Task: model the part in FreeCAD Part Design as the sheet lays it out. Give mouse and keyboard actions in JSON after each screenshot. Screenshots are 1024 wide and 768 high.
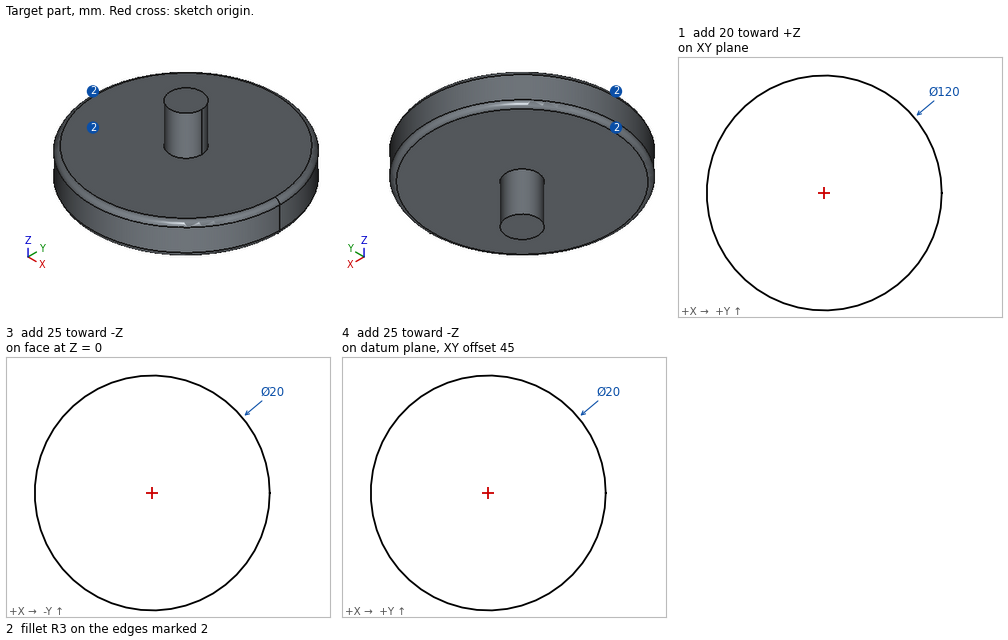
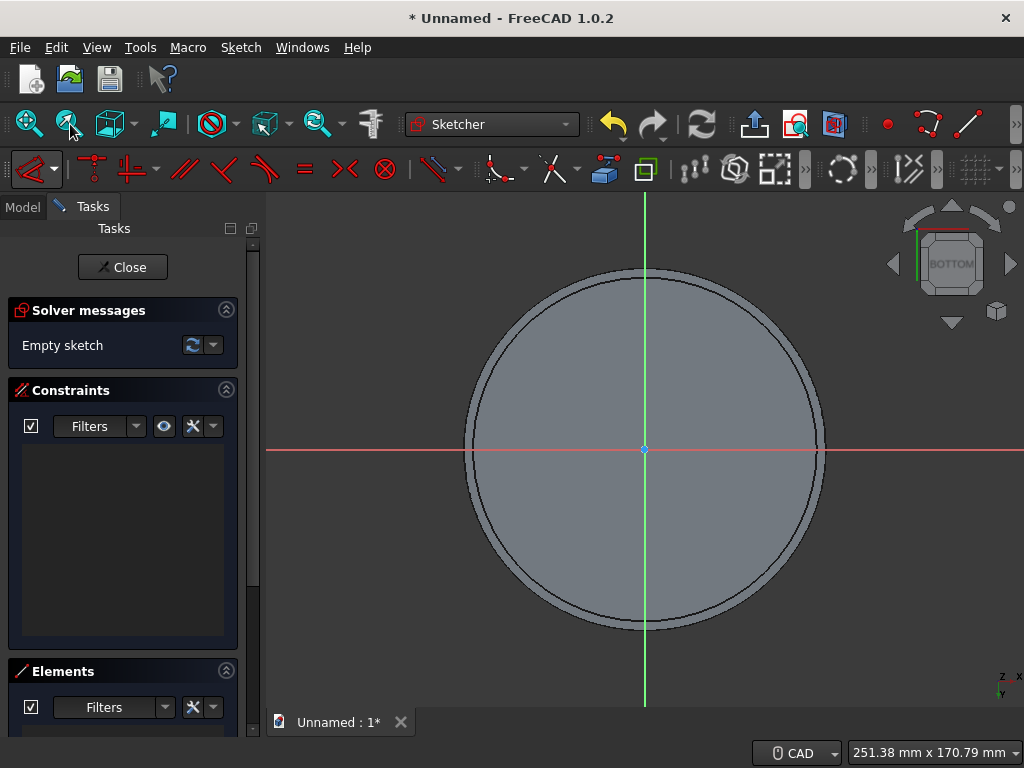
{"action": "scroll", "coordinate": [662, 449], "scroll_direction": "up", "scroll_amount": 8}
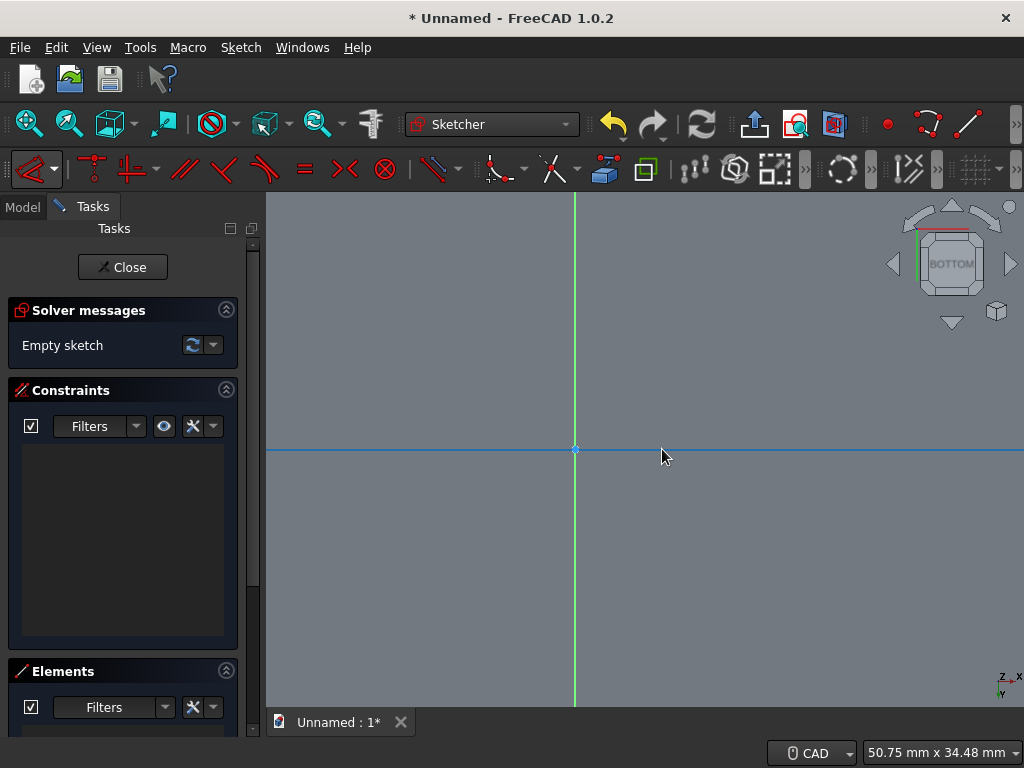
{"action": "key", "text": "g c"}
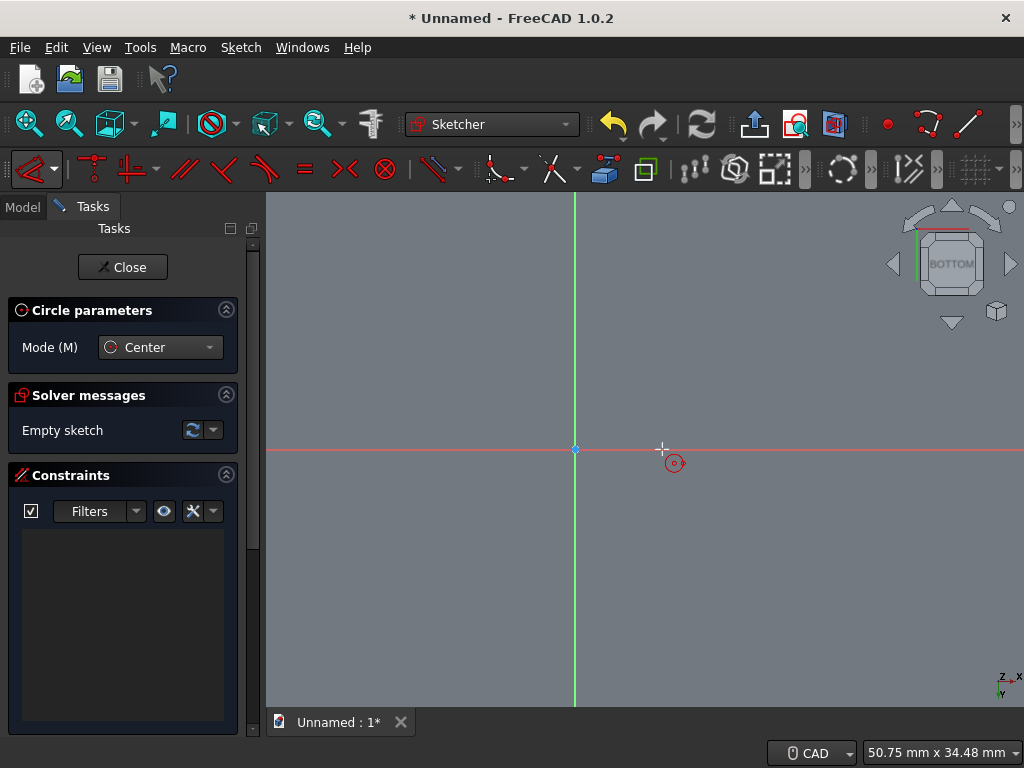
{"action": "left_click", "coordinate": [575, 450]}
{"action": "left_click", "coordinate": [681, 344]}
{"action": "key", "text": "Escape"}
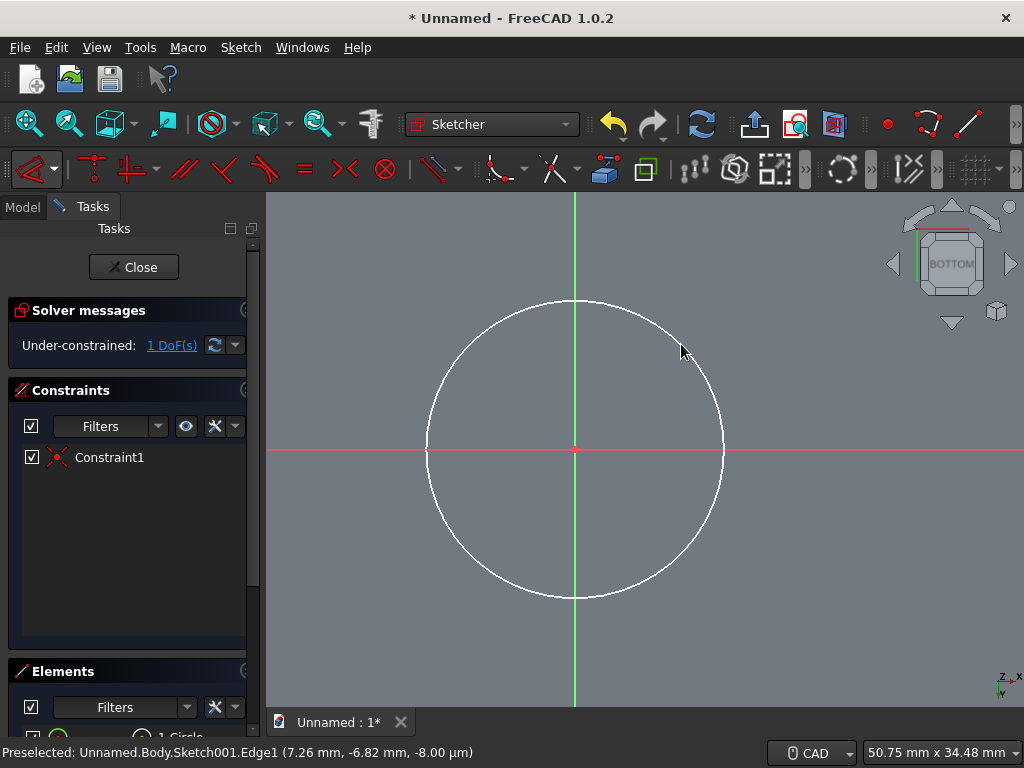
{"action": "left_click", "coordinate": [680, 344]}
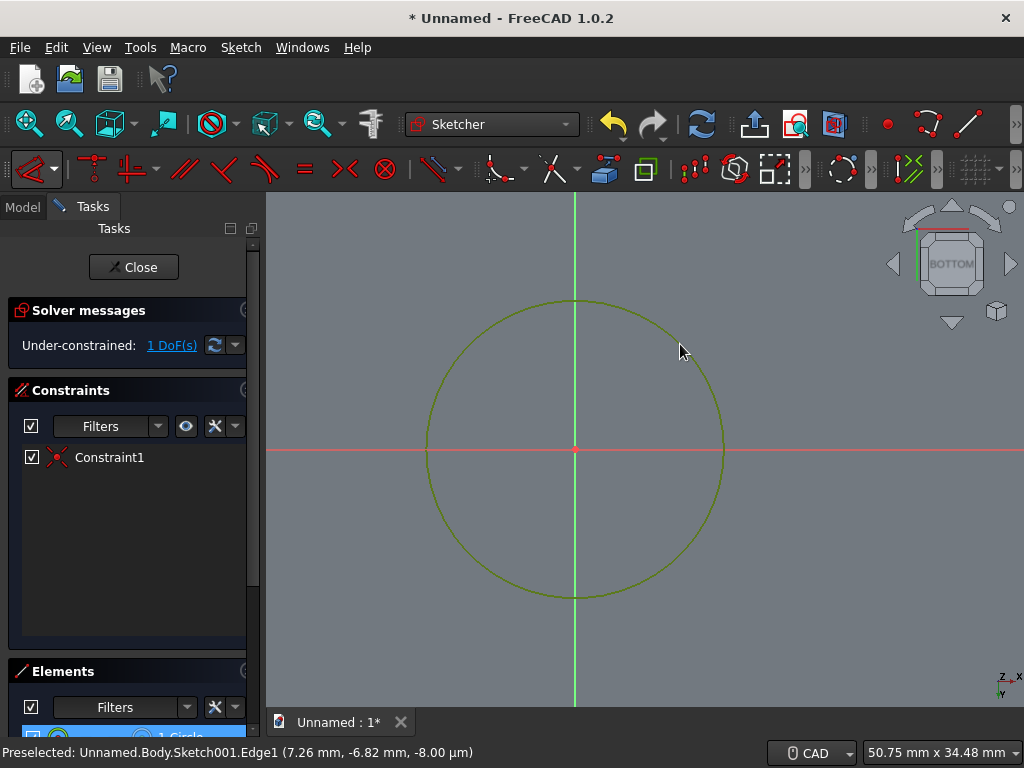
{"action": "key", "text": "k o"}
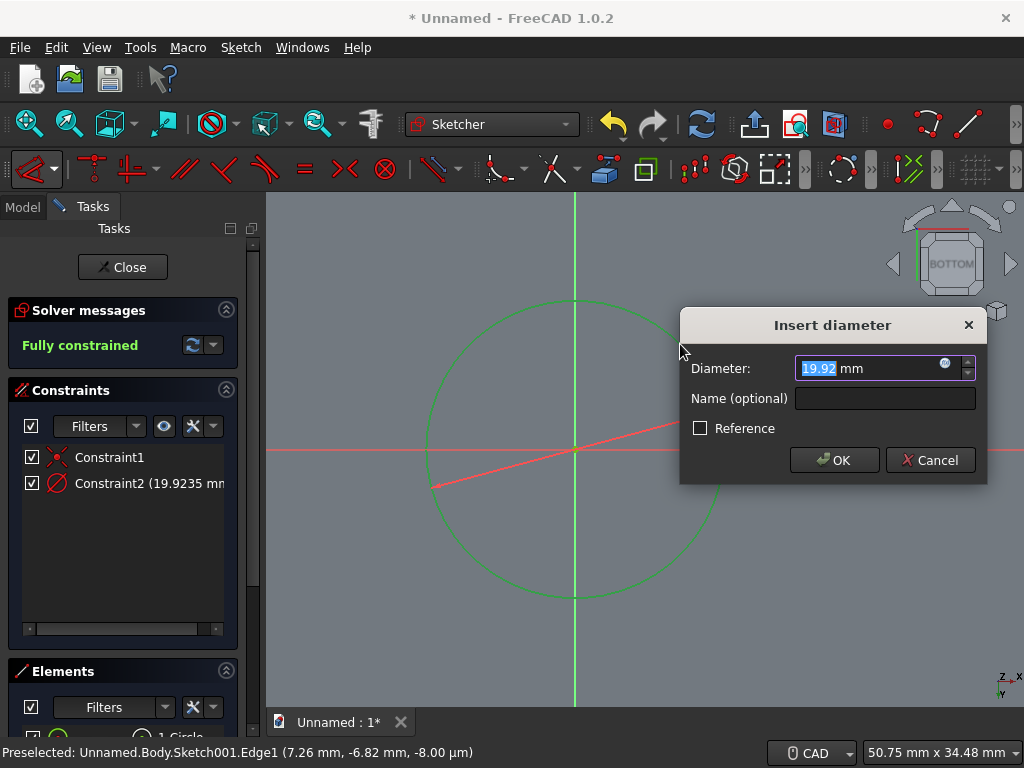
{"action": "type", "text": "20"}
{"action": "key", "text": "Return"}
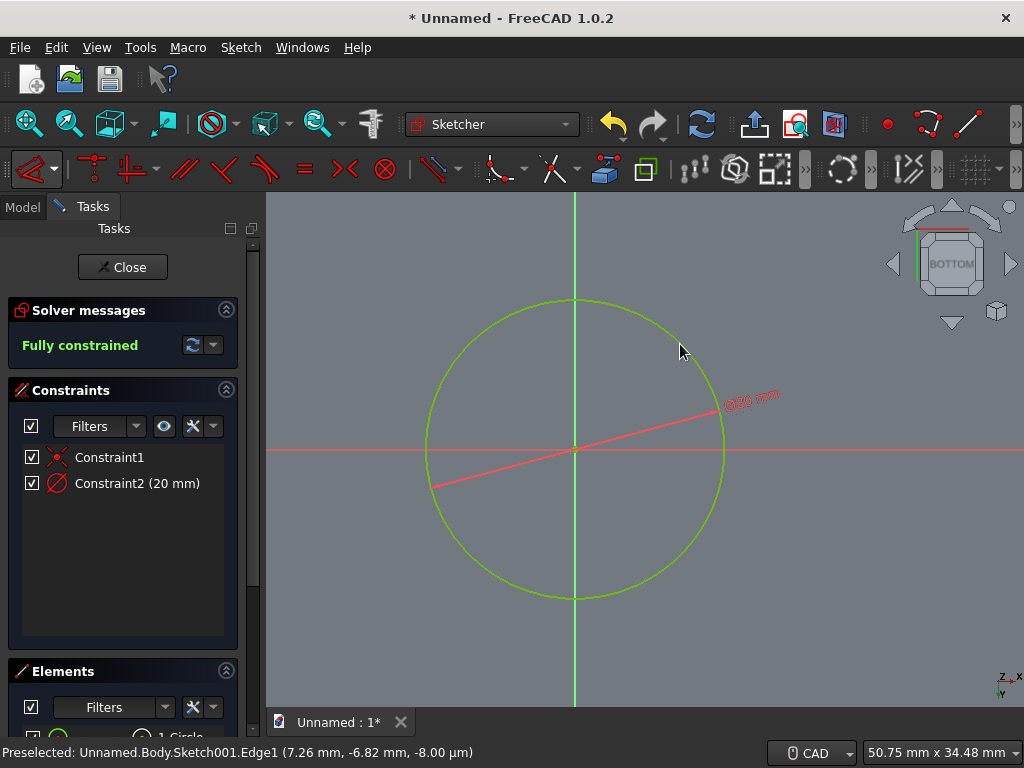
{"action": "left_click", "coordinate": [123, 267]}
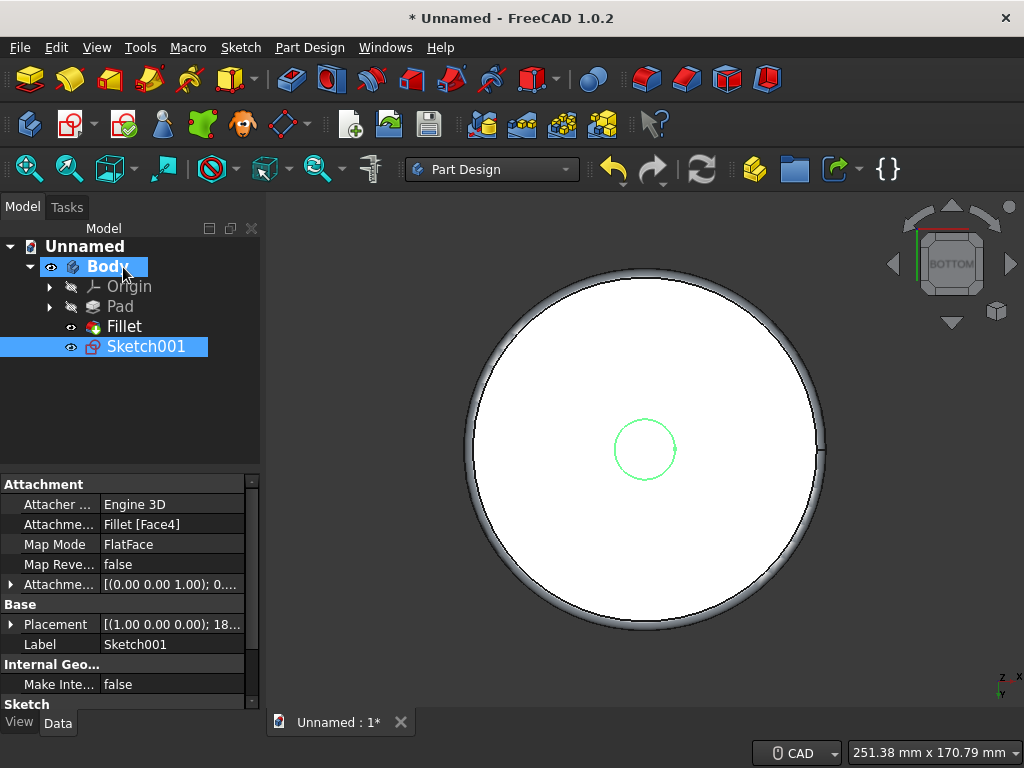
{"action": "left_click", "coordinate": [30, 80]}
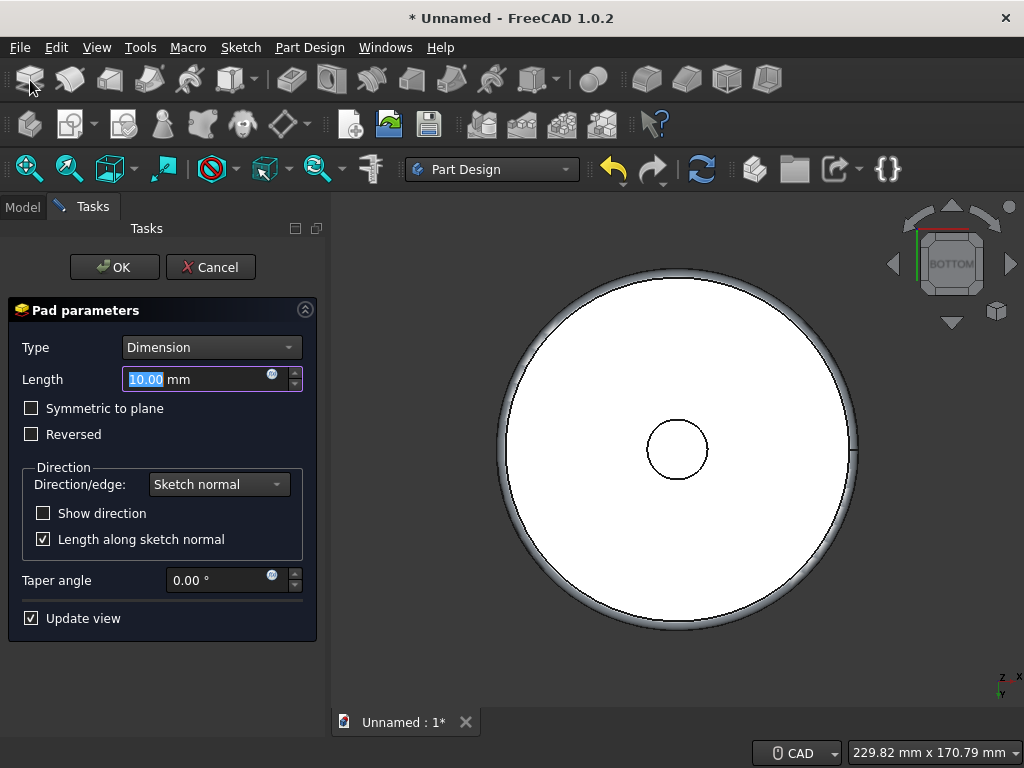
{"action": "type", "text": "25"}
{"action": "key", "text": "Tab"}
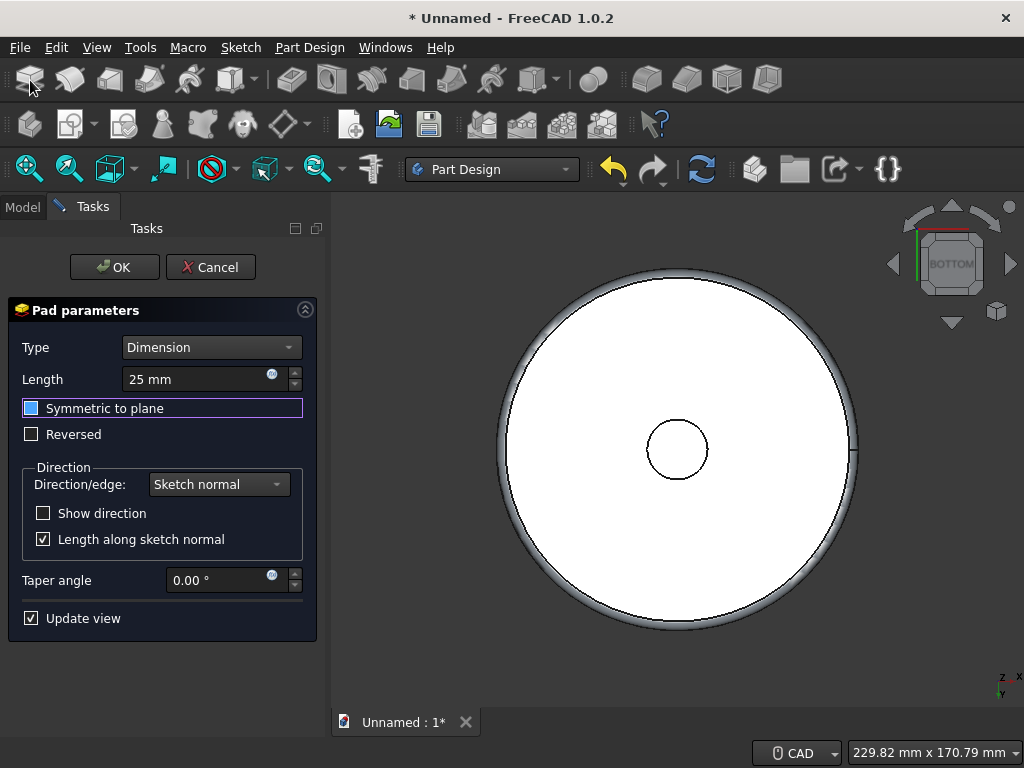
{"action": "left_click", "coordinate": [115, 267]}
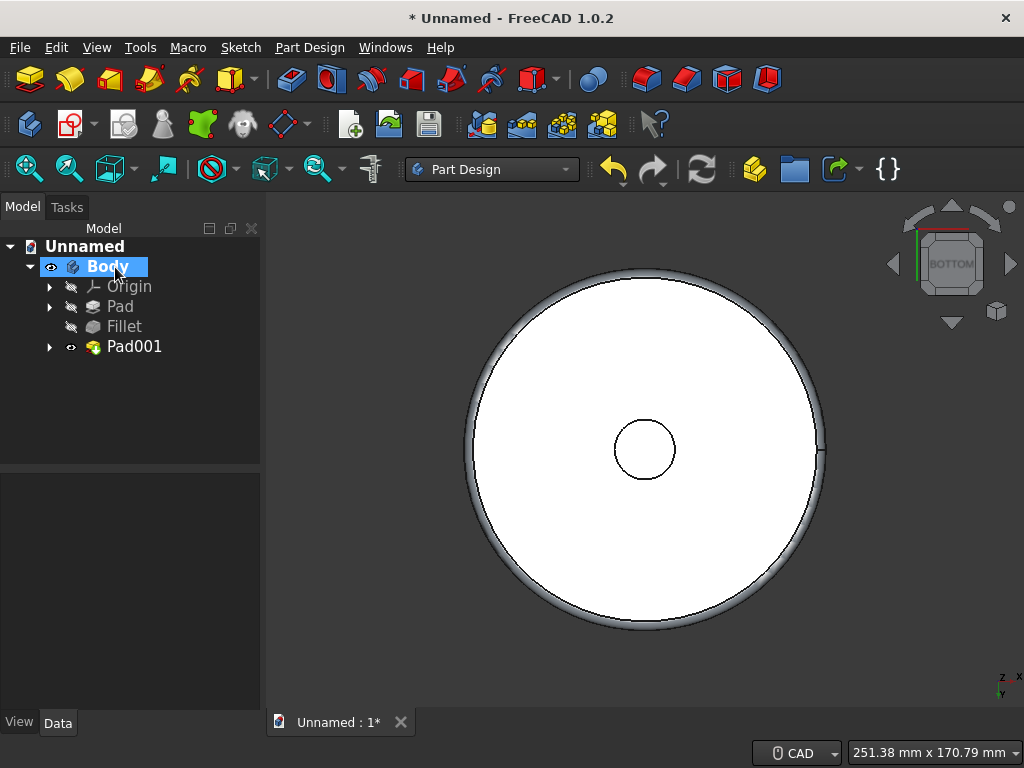
{"action": "left_click", "coordinate": [50, 287]}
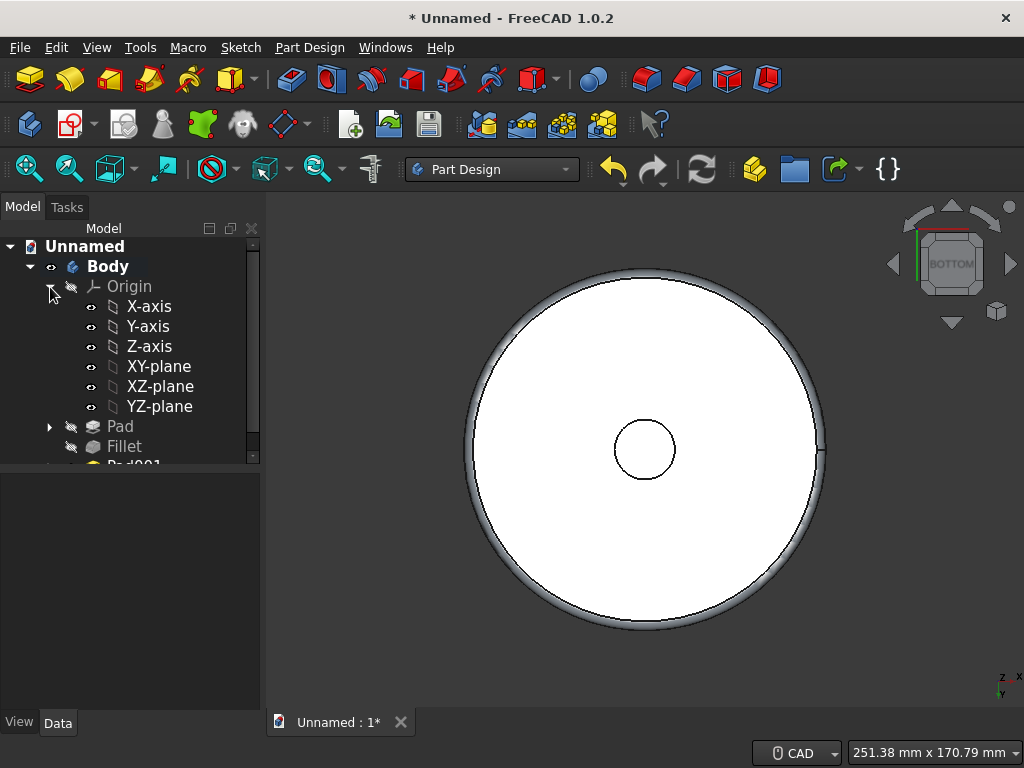
{"action": "left_click", "coordinate": [136, 367]}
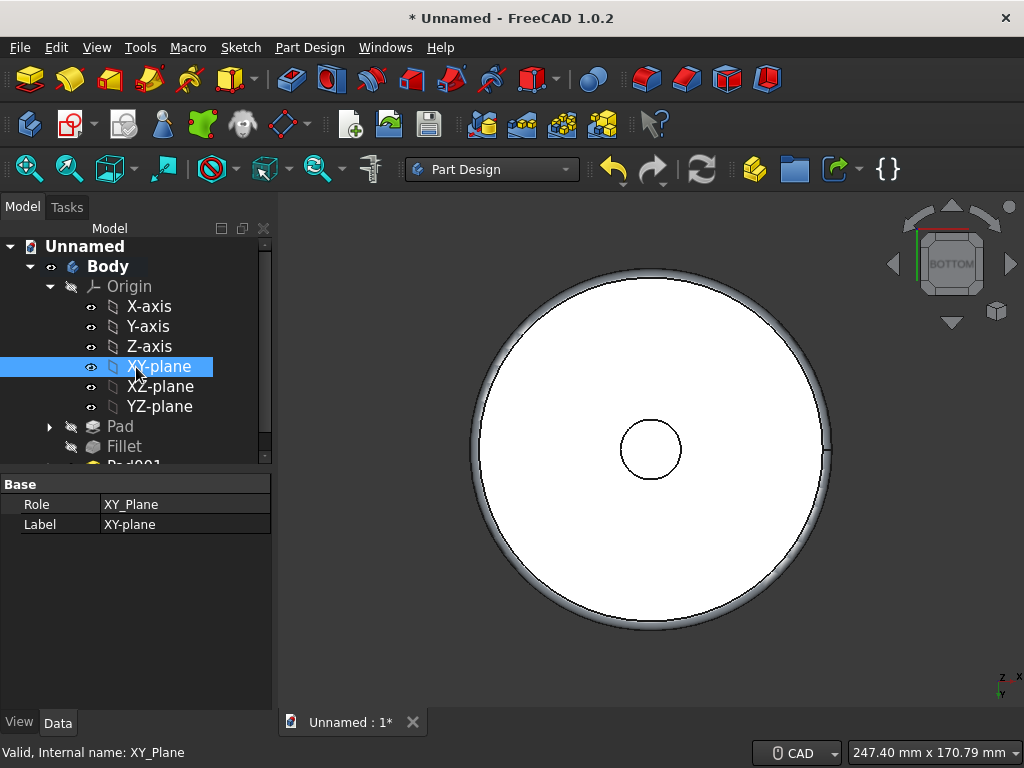
{"action": "left_click", "coordinate": [284, 124]}